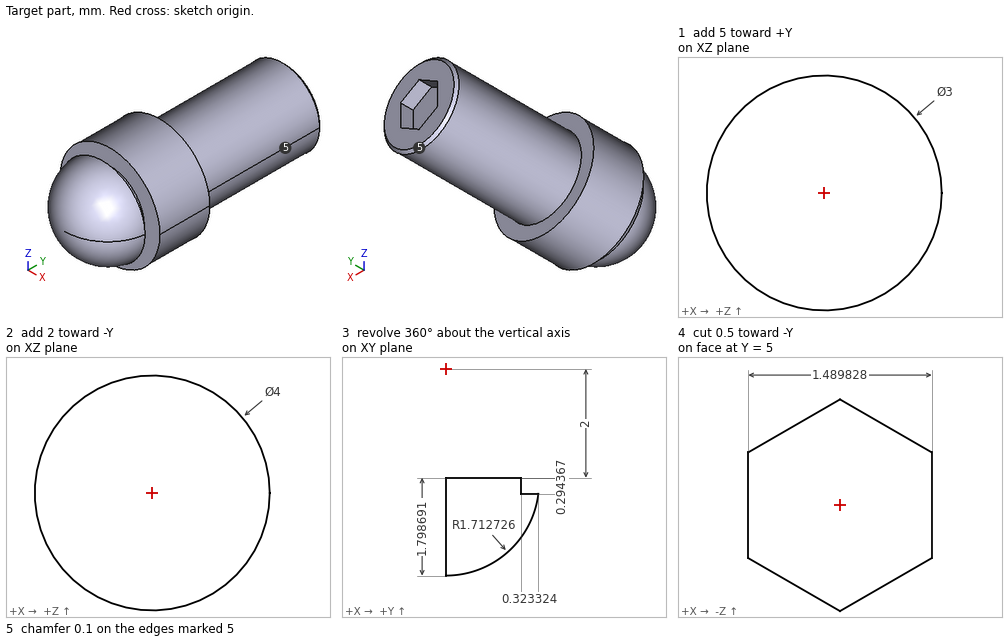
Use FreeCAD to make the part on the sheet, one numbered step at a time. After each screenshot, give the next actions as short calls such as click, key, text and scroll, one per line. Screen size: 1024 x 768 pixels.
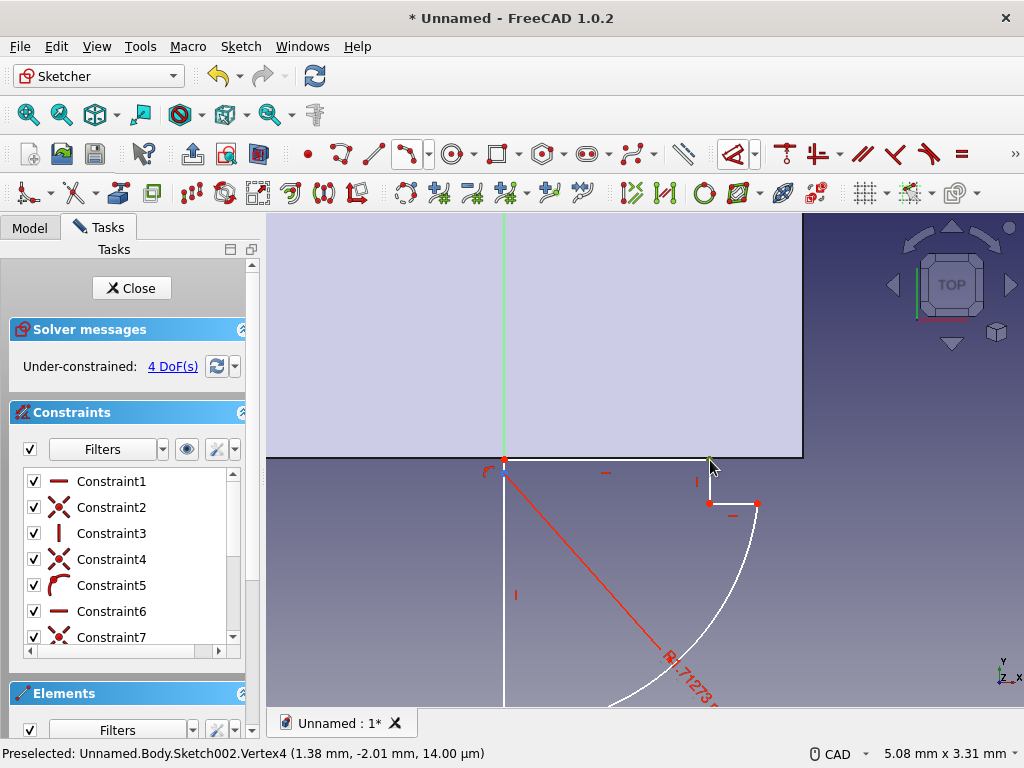
click(754, 154)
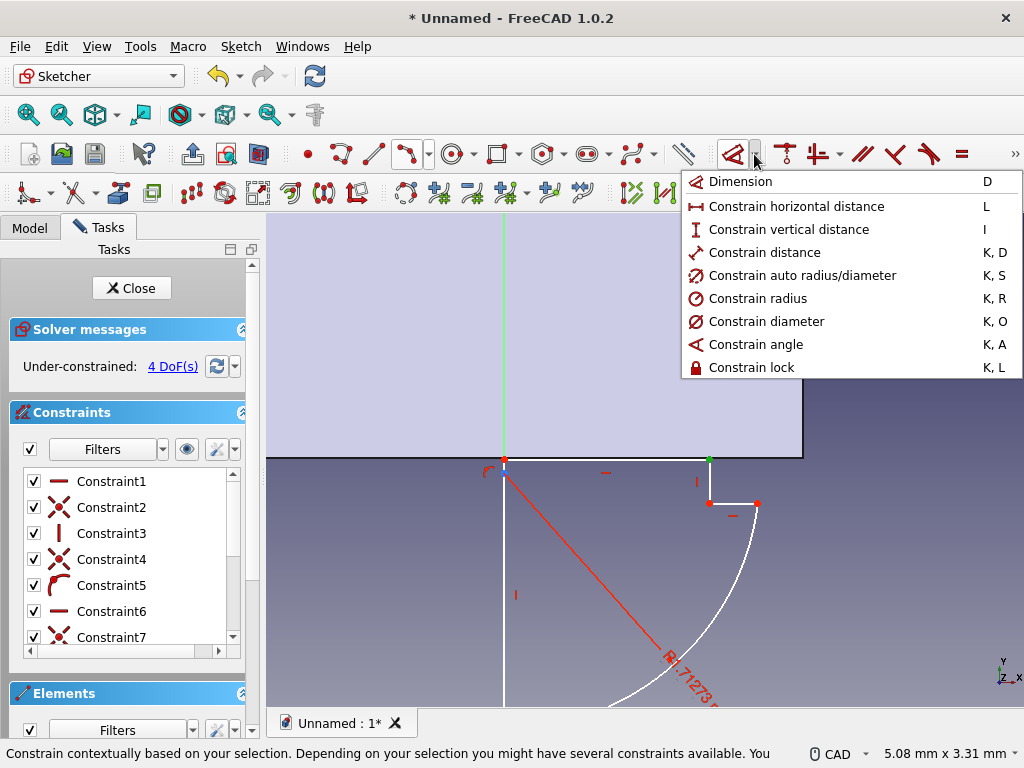
click(852, 230)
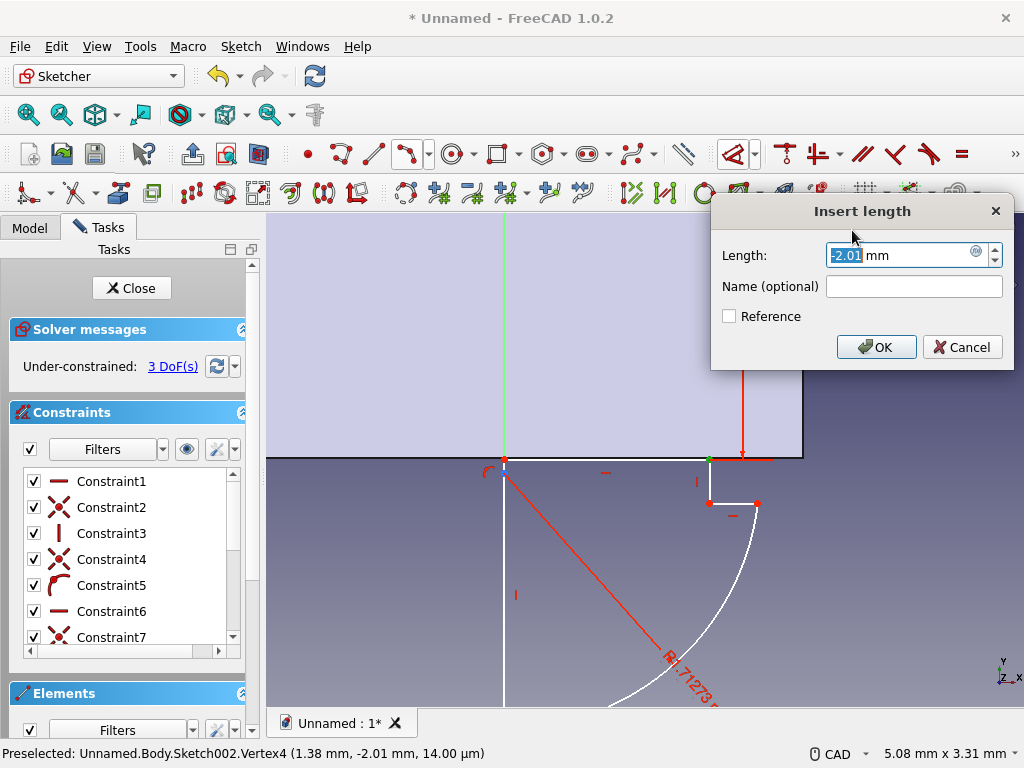
text(-2)
key(Return)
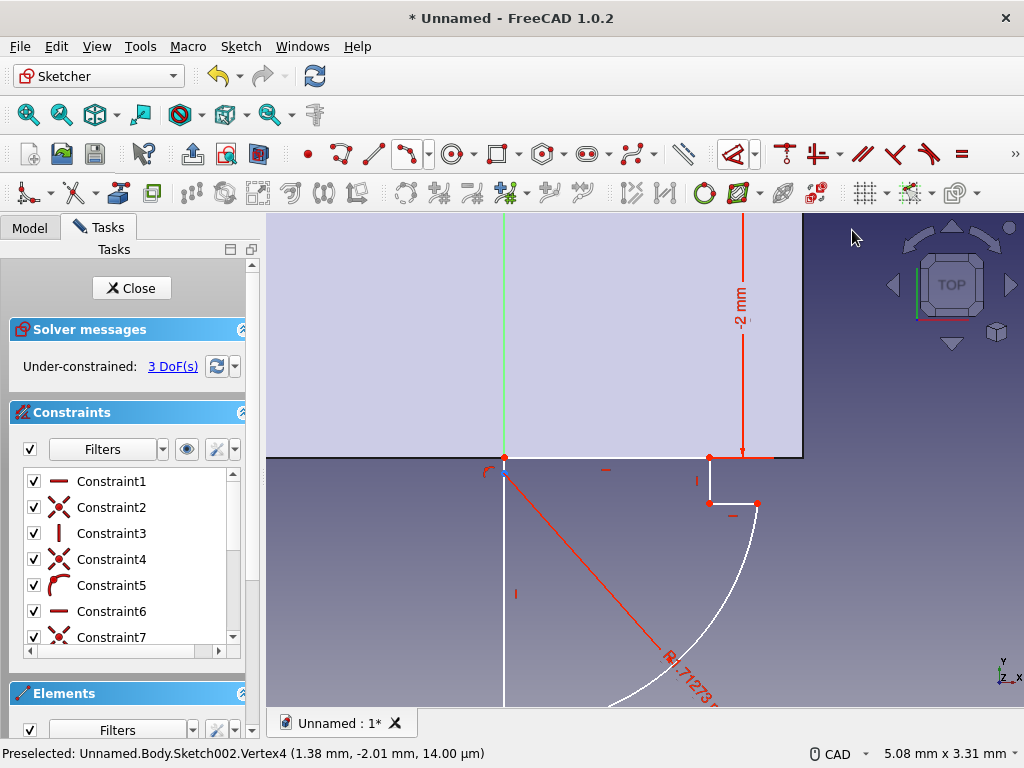
click(743, 504)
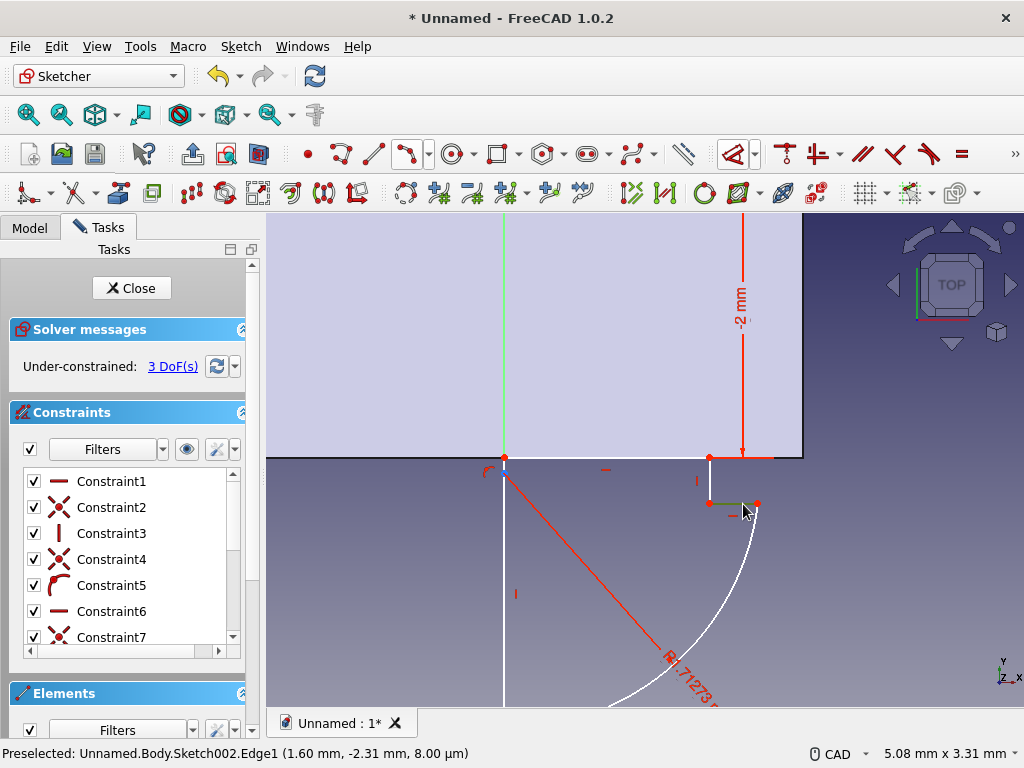
click(754, 154)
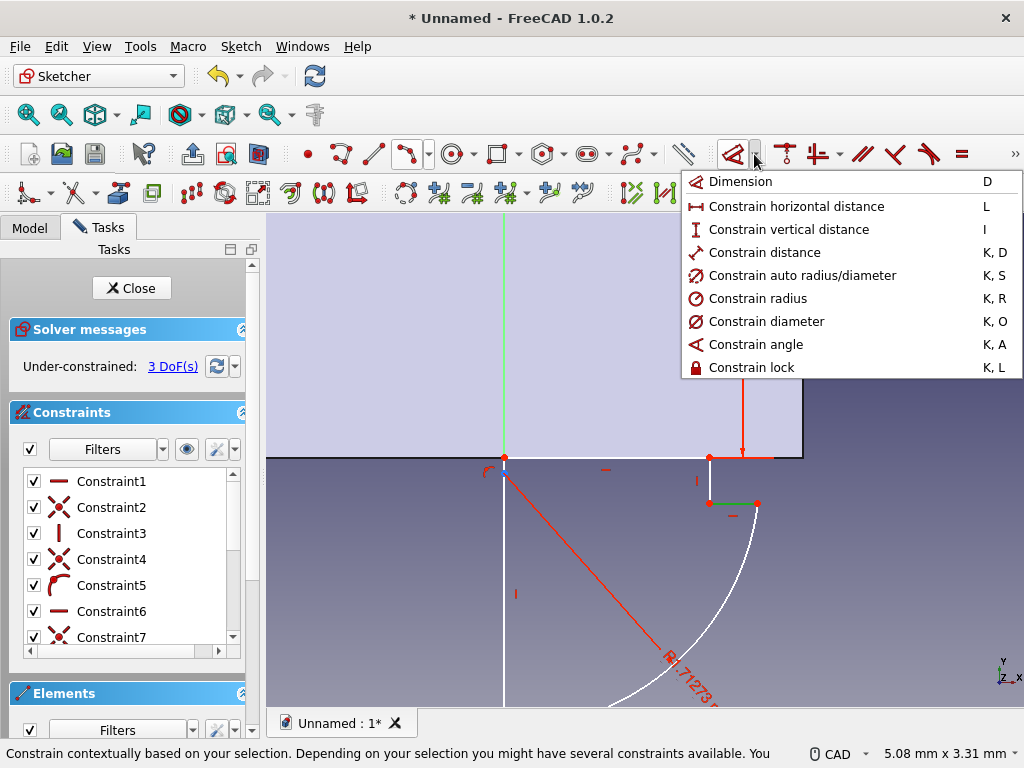
click(852, 206)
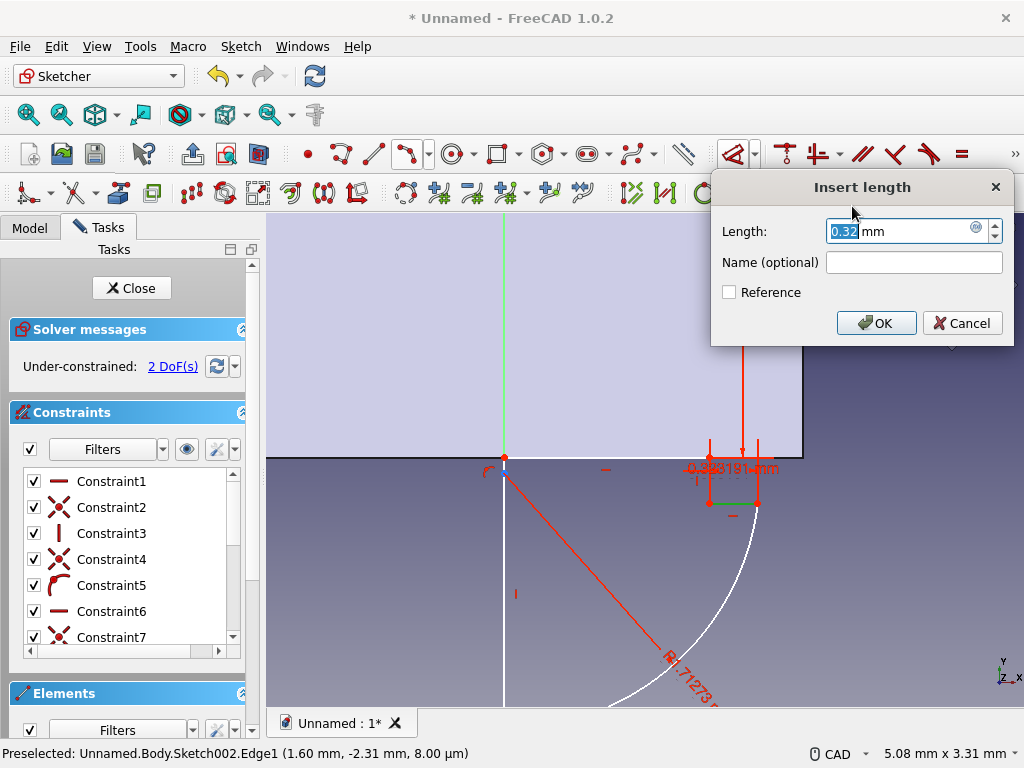
text(0.323324)
key(Return)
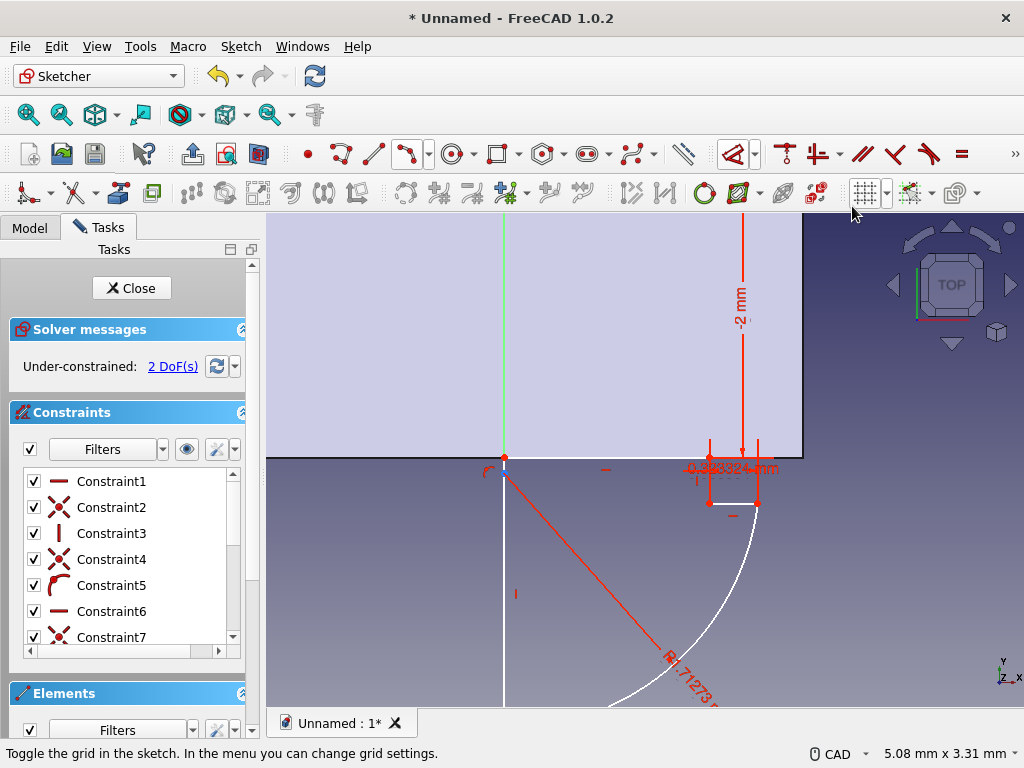
click(710, 490)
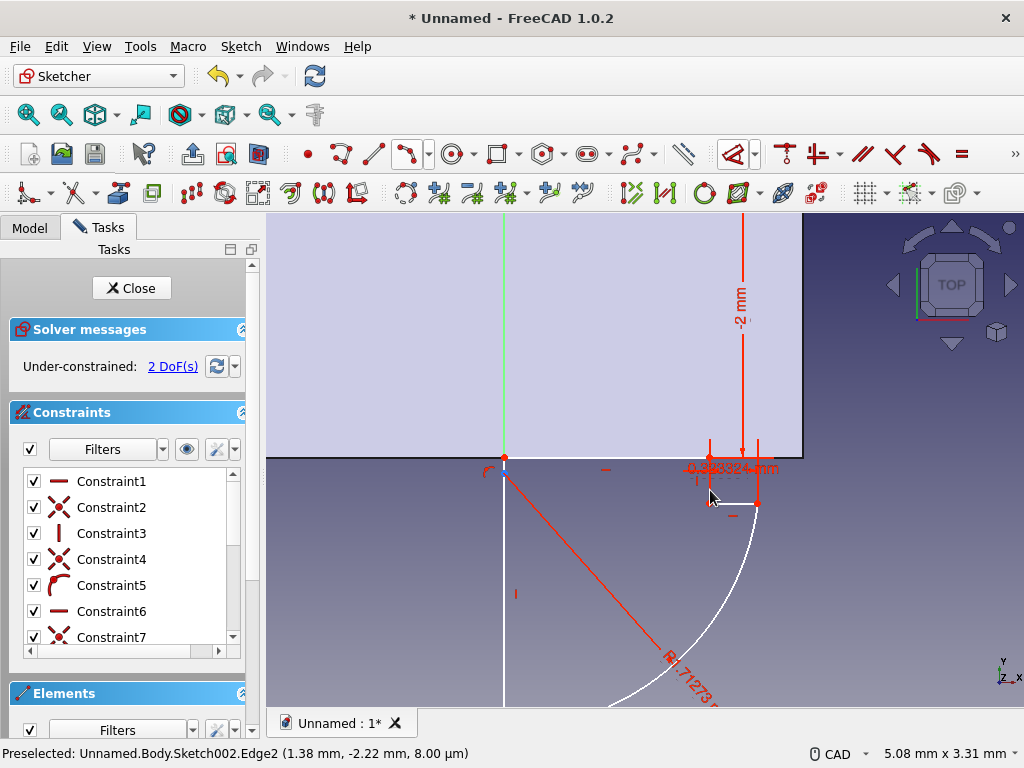
key(i)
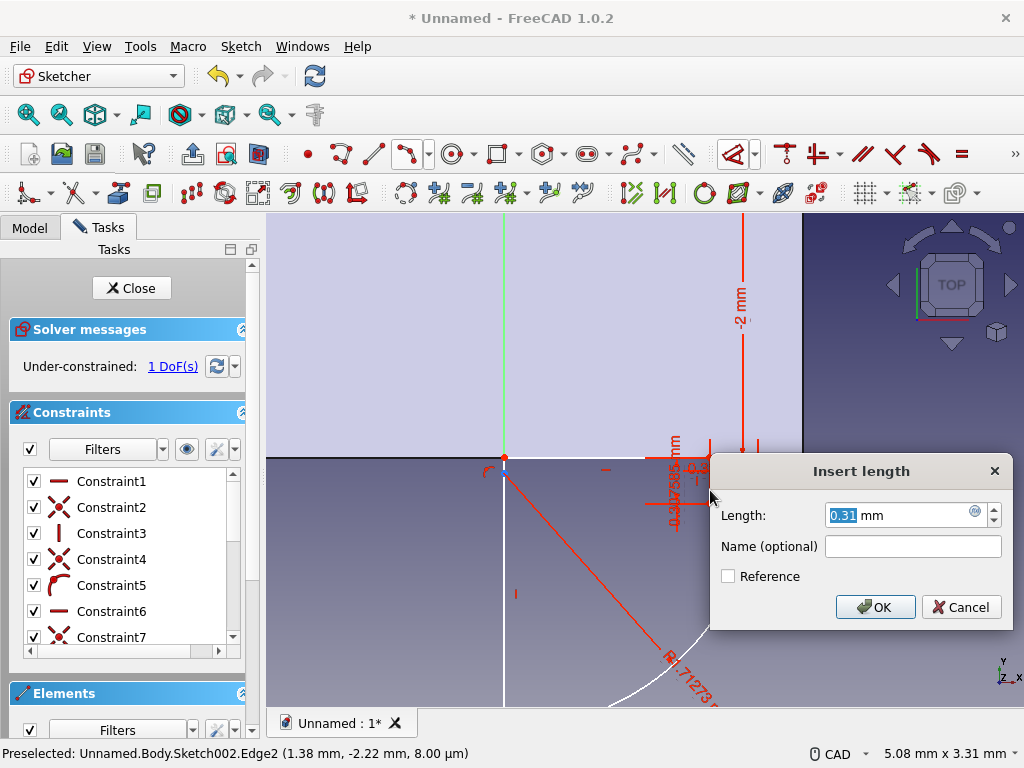
text(0.294367)
key(Return)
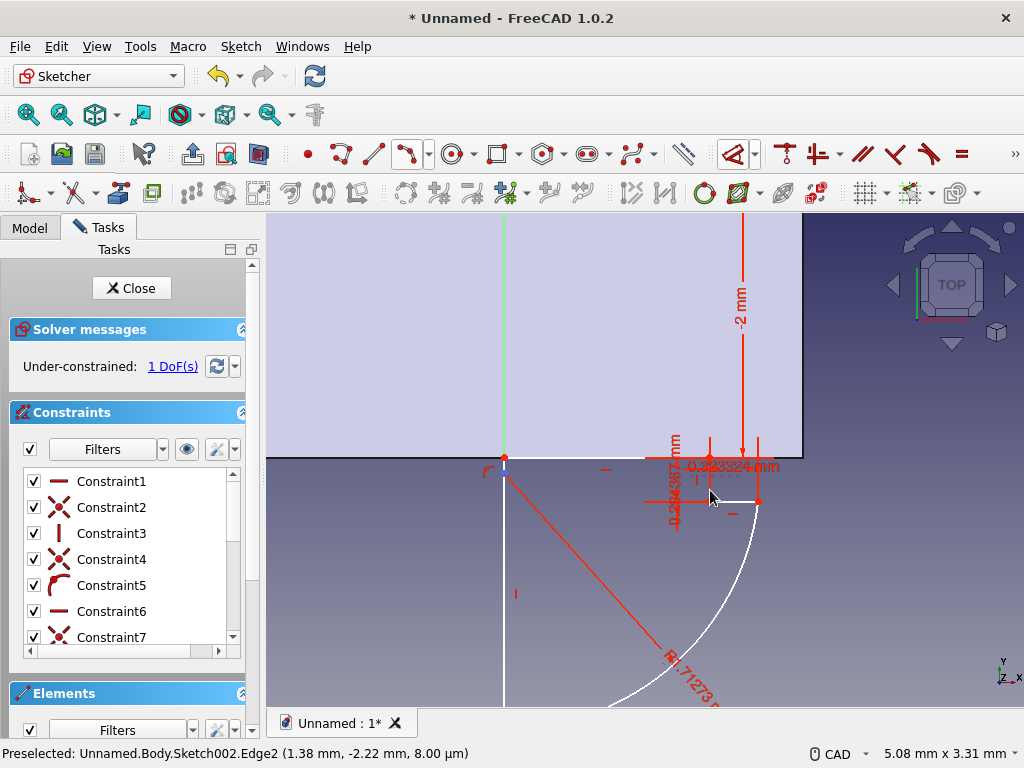
click(504, 539)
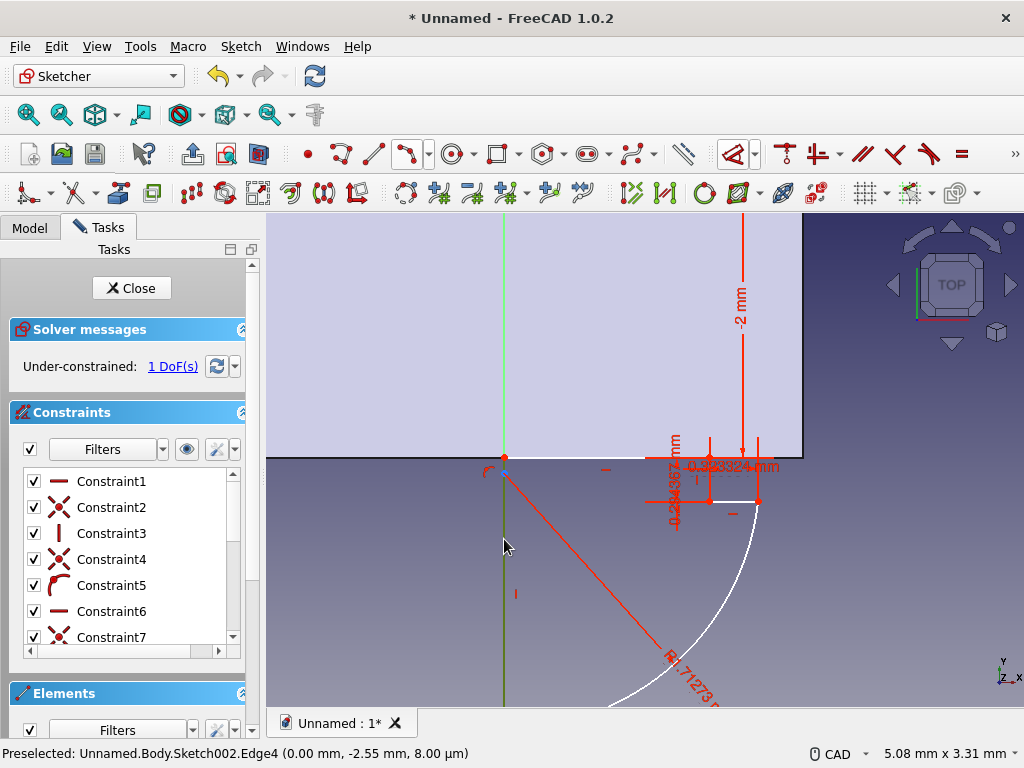
click(754, 154)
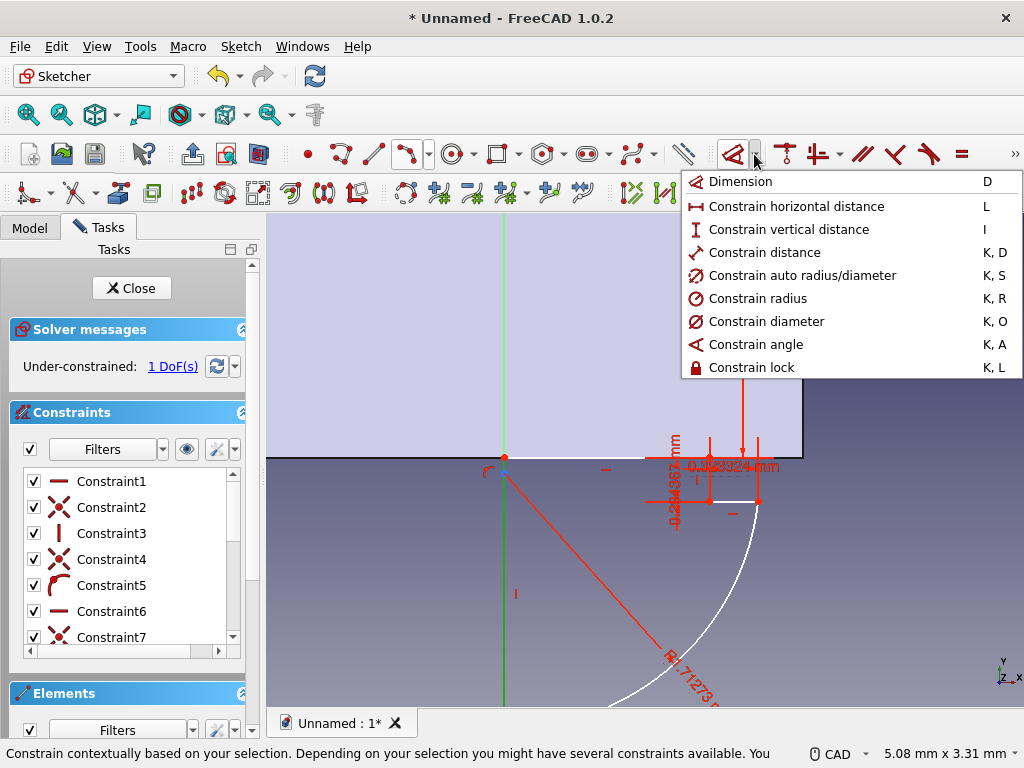
click(852, 230)